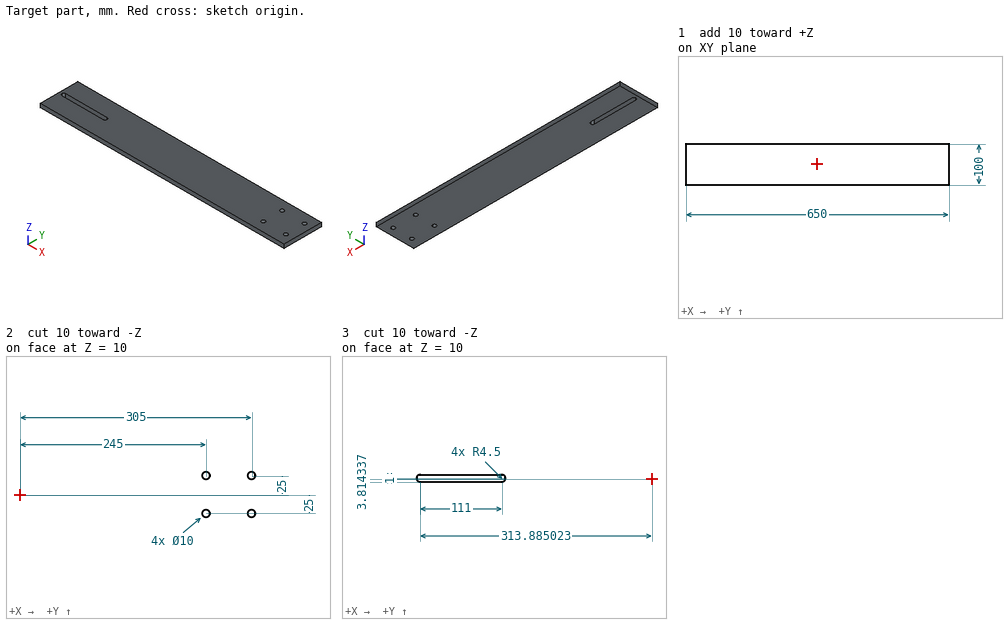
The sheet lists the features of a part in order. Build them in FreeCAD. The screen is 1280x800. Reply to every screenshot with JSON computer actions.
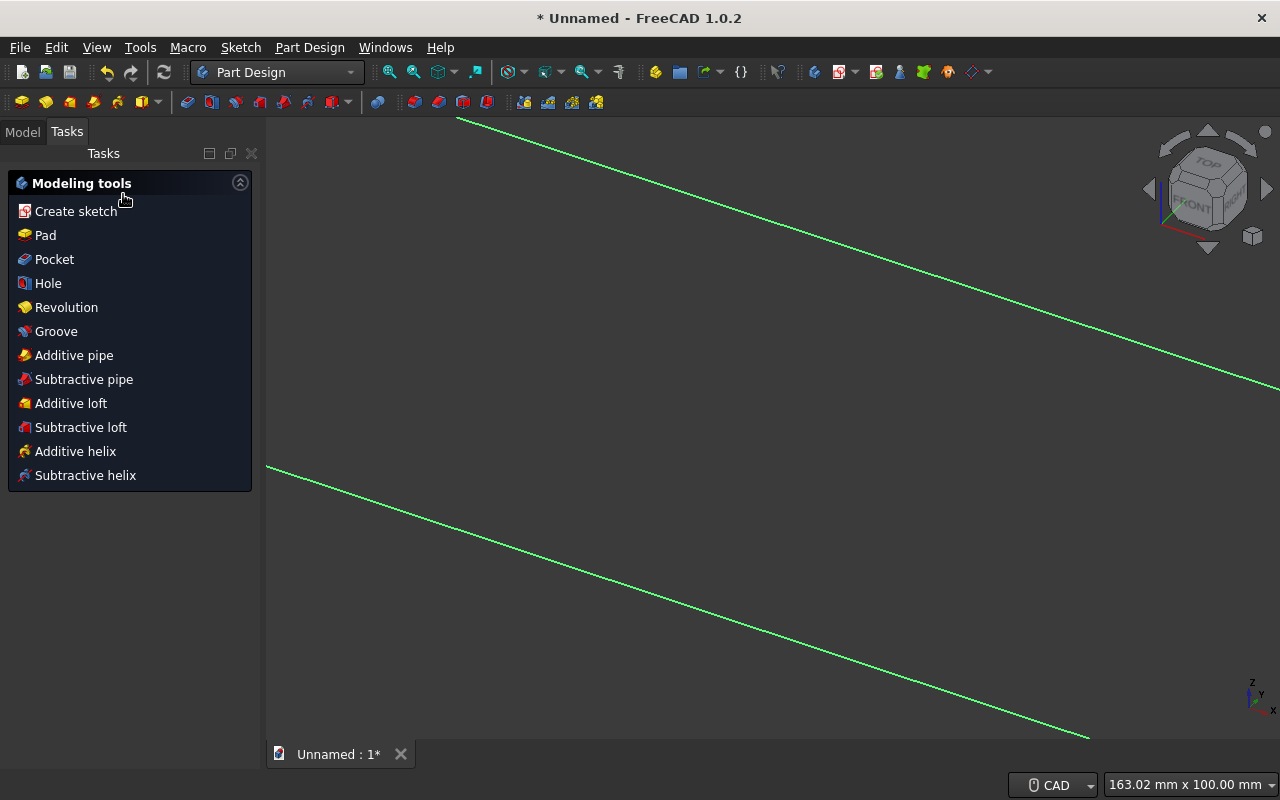
{"action": "left_click", "coordinate": [22, 102]}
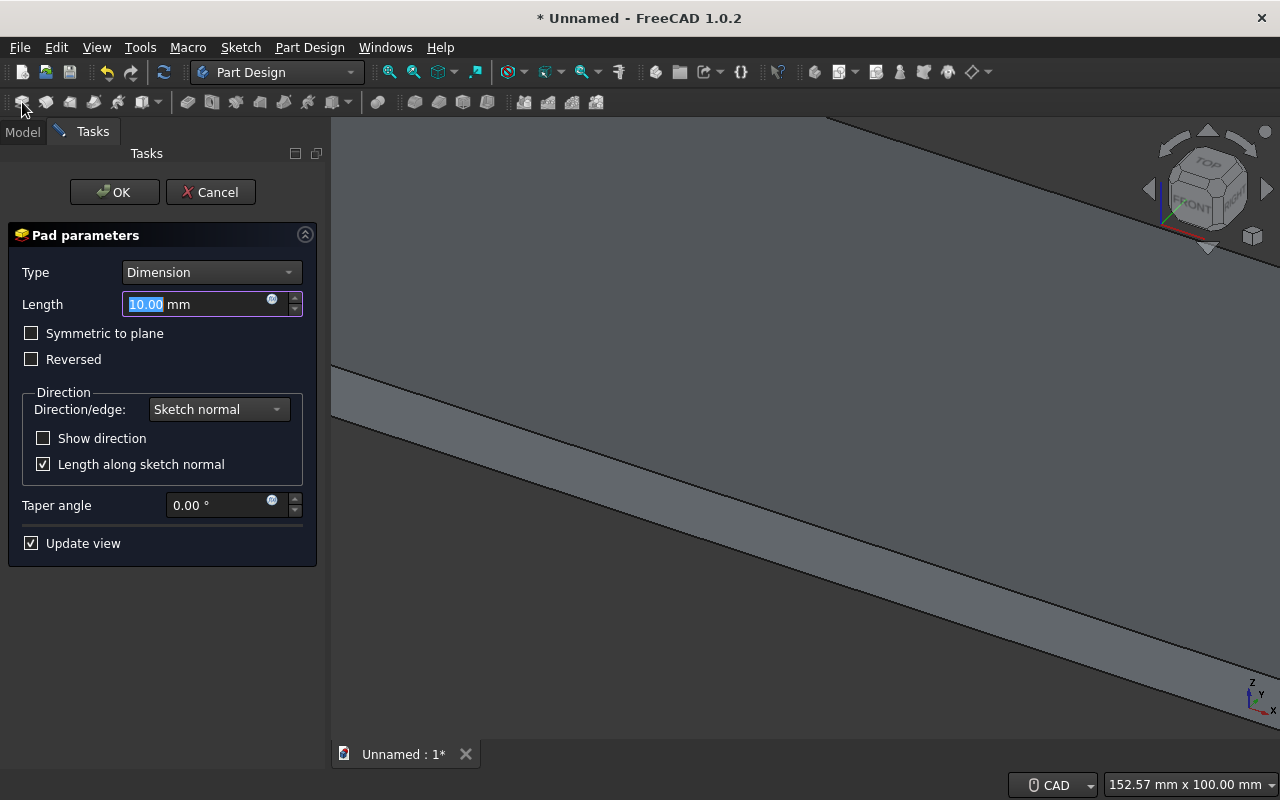
{"action": "type", "text": "10"}
{"action": "key", "text": "Tab"}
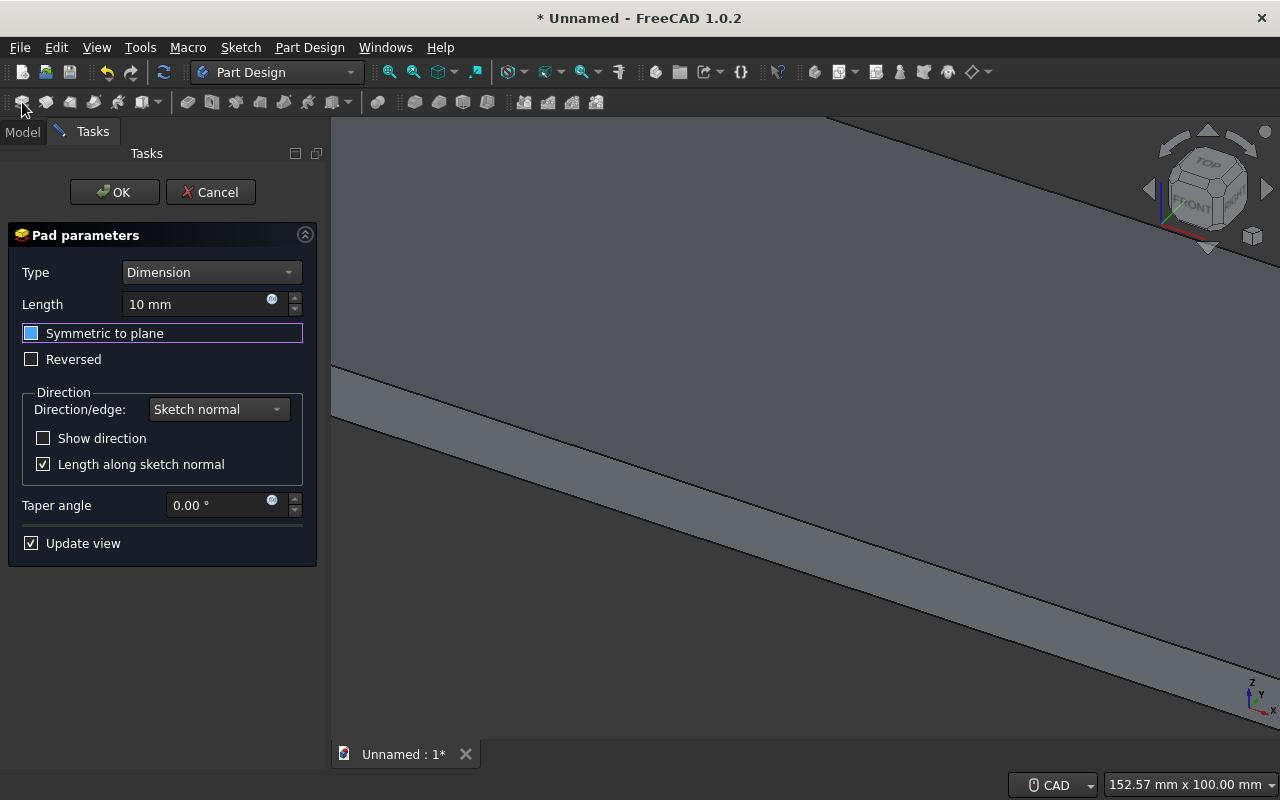
{"action": "left_click", "coordinate": [115, 192]}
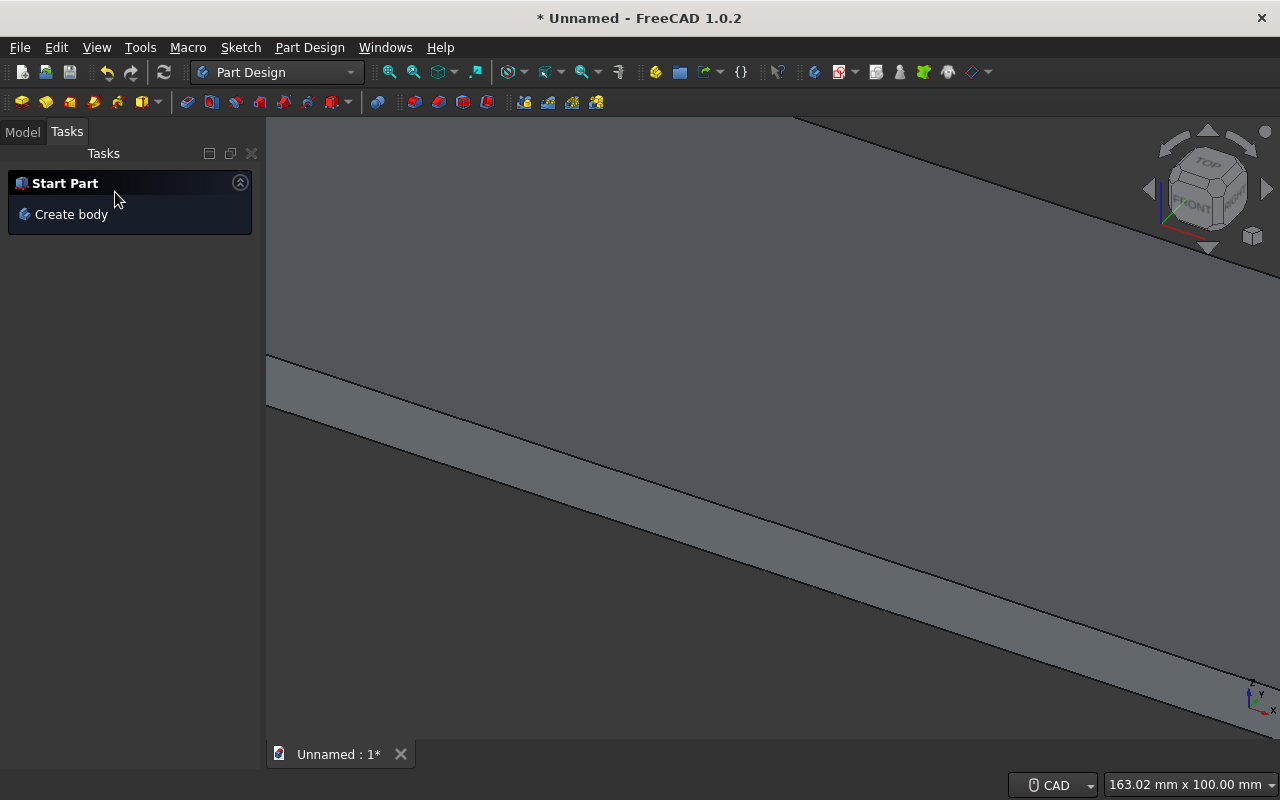
{"action": "key", "text": "v f"}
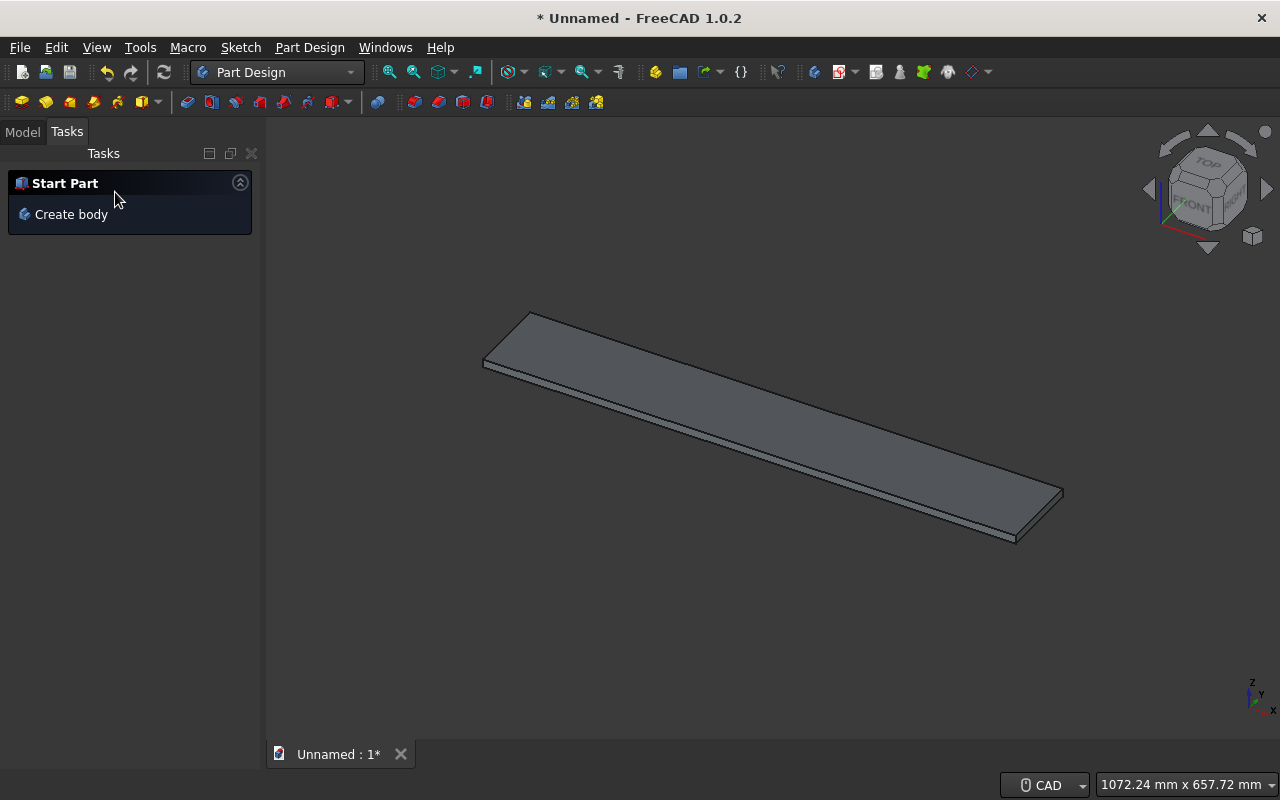
{"action": "left_click", "coordinate": [925, 473]}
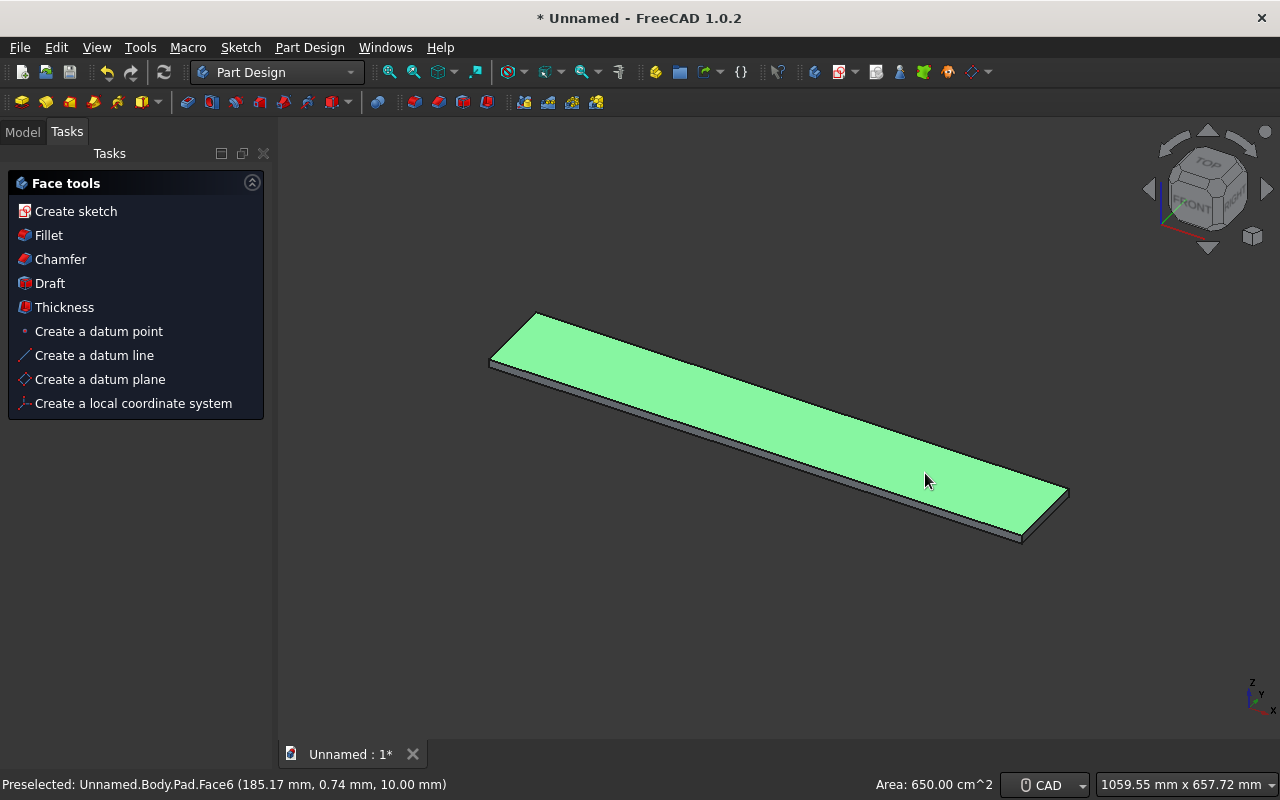
{"action": "left_click", "coordinate": [840, 72]}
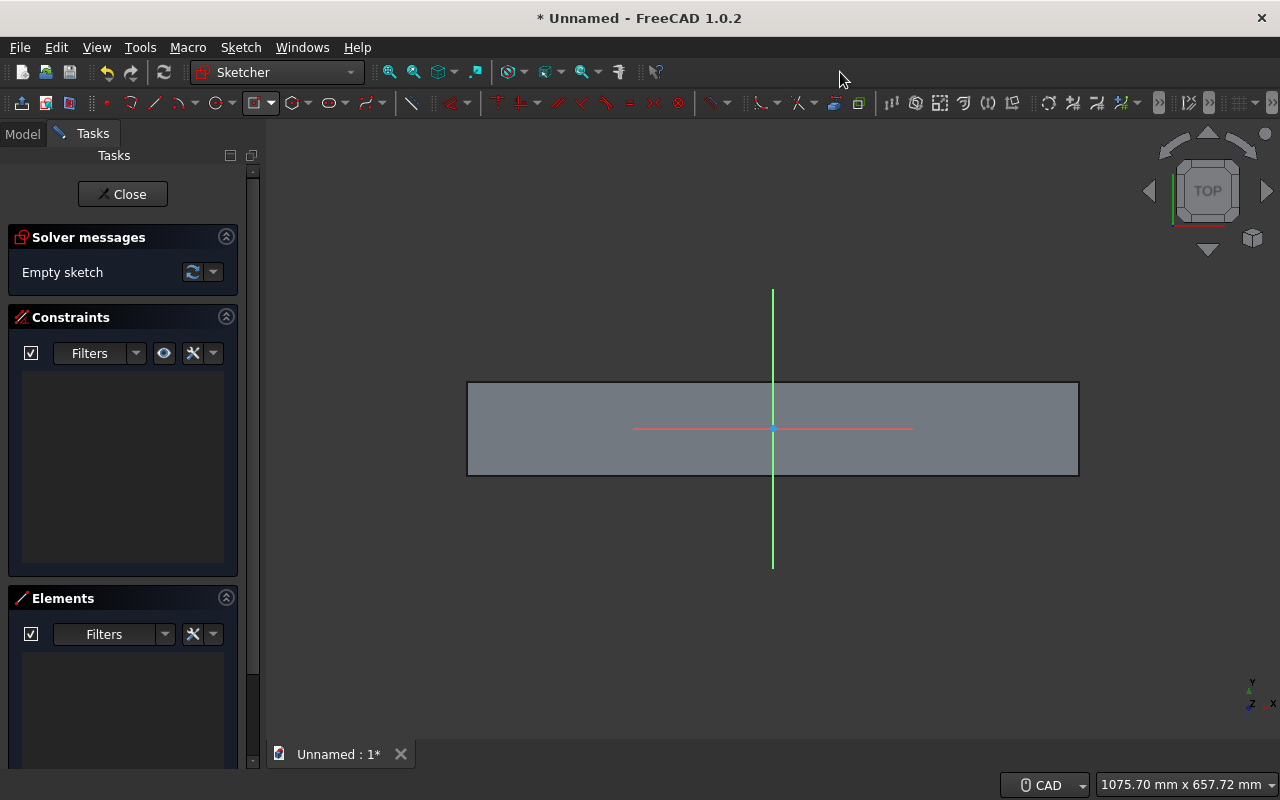
{"action": "scroll", "coordinate": [1084, 429], "scroll_direction": "up", "scroll_amount": 10}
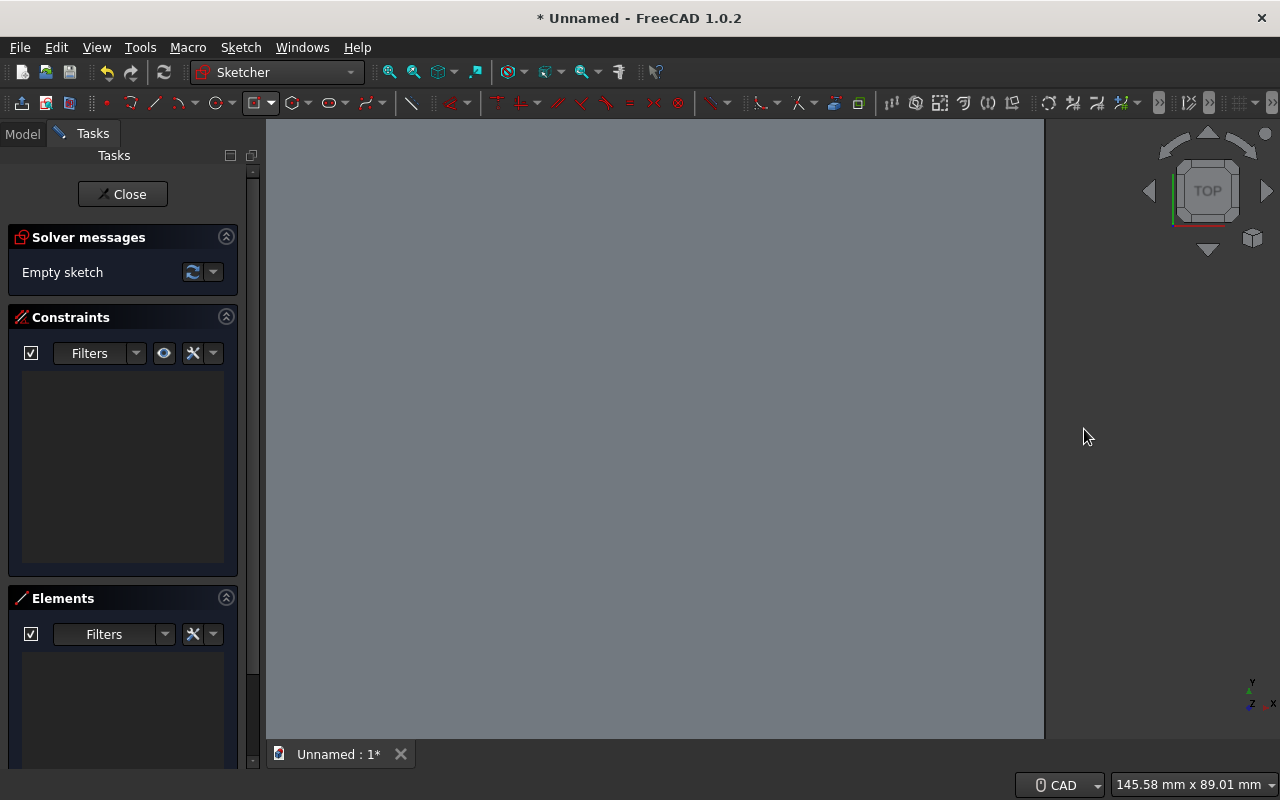
{"action": "key", "text": "g c"}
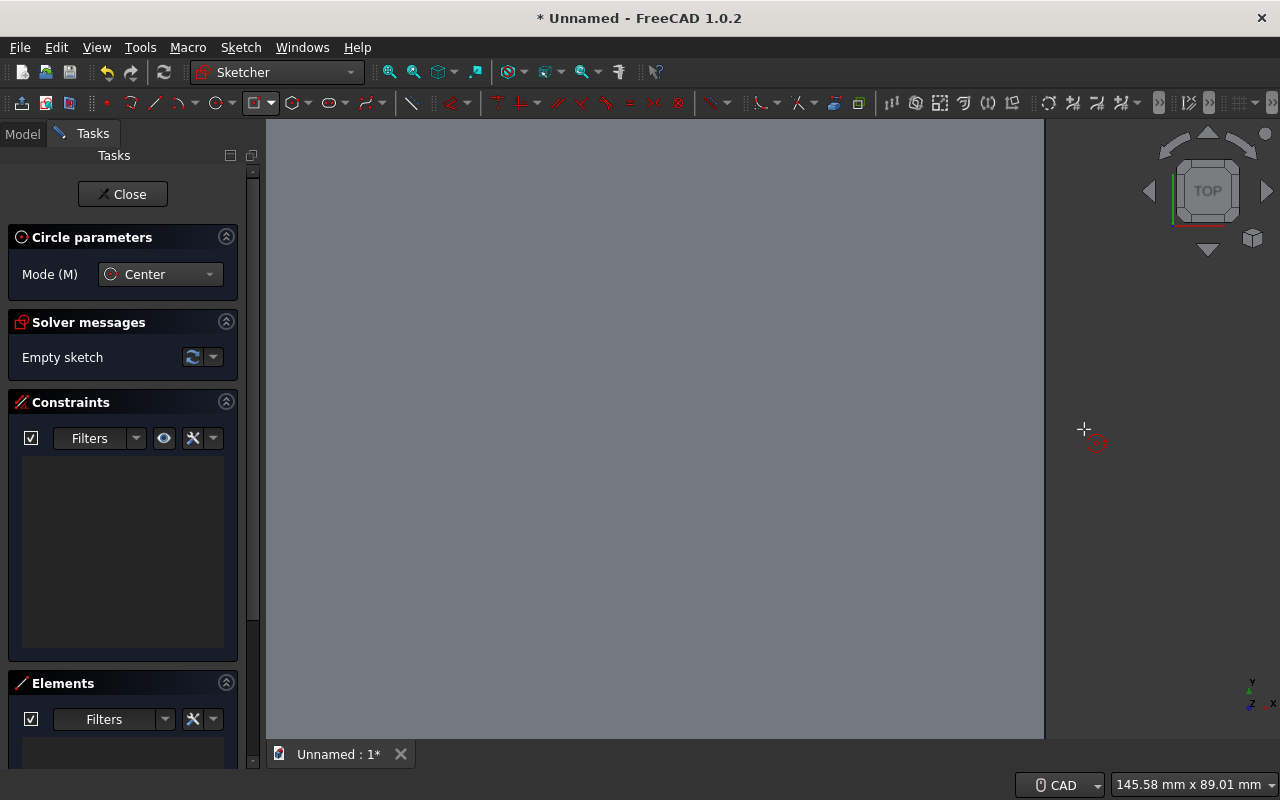
{"action": "left_click", "coordinate": [905, 252]}
{"action": "mouse_move", "coordinate": [930, 227]}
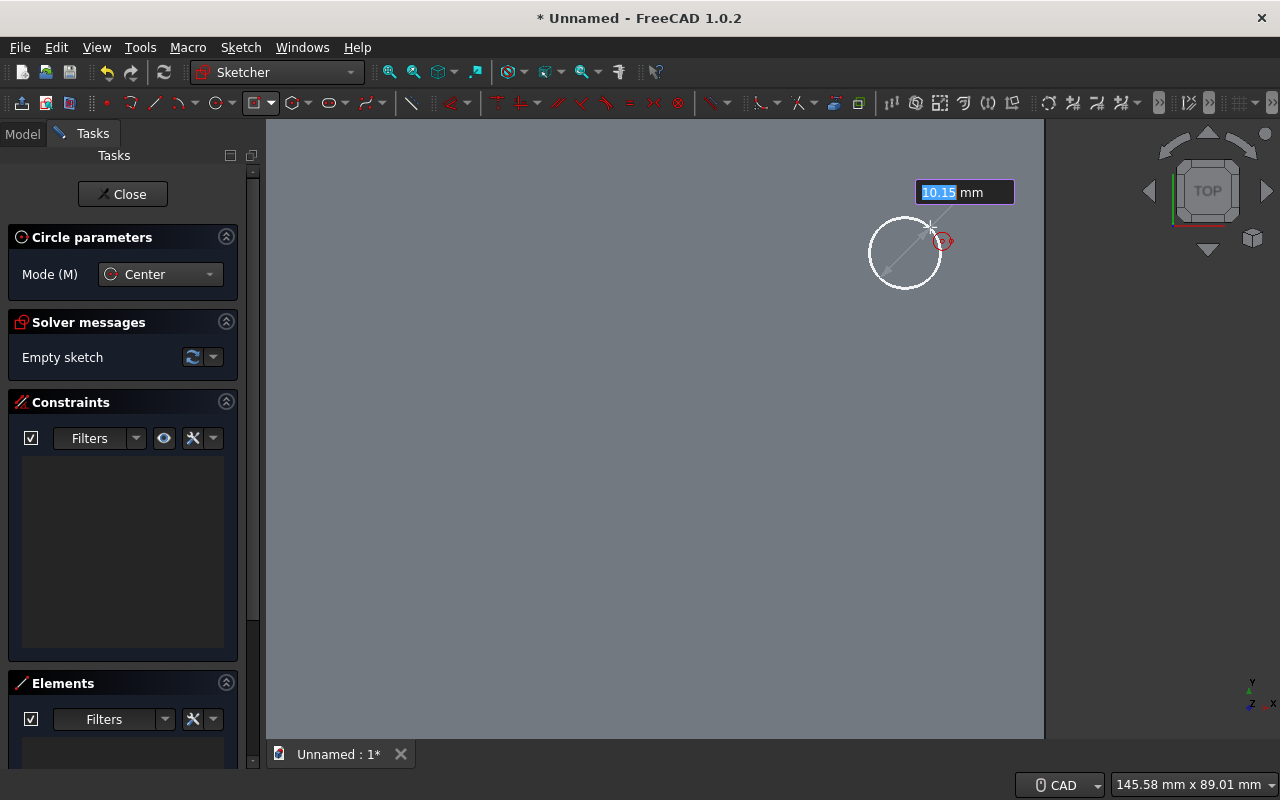
{"action": "type", "text": "10"}
{"action": "key", "text": "Return"}